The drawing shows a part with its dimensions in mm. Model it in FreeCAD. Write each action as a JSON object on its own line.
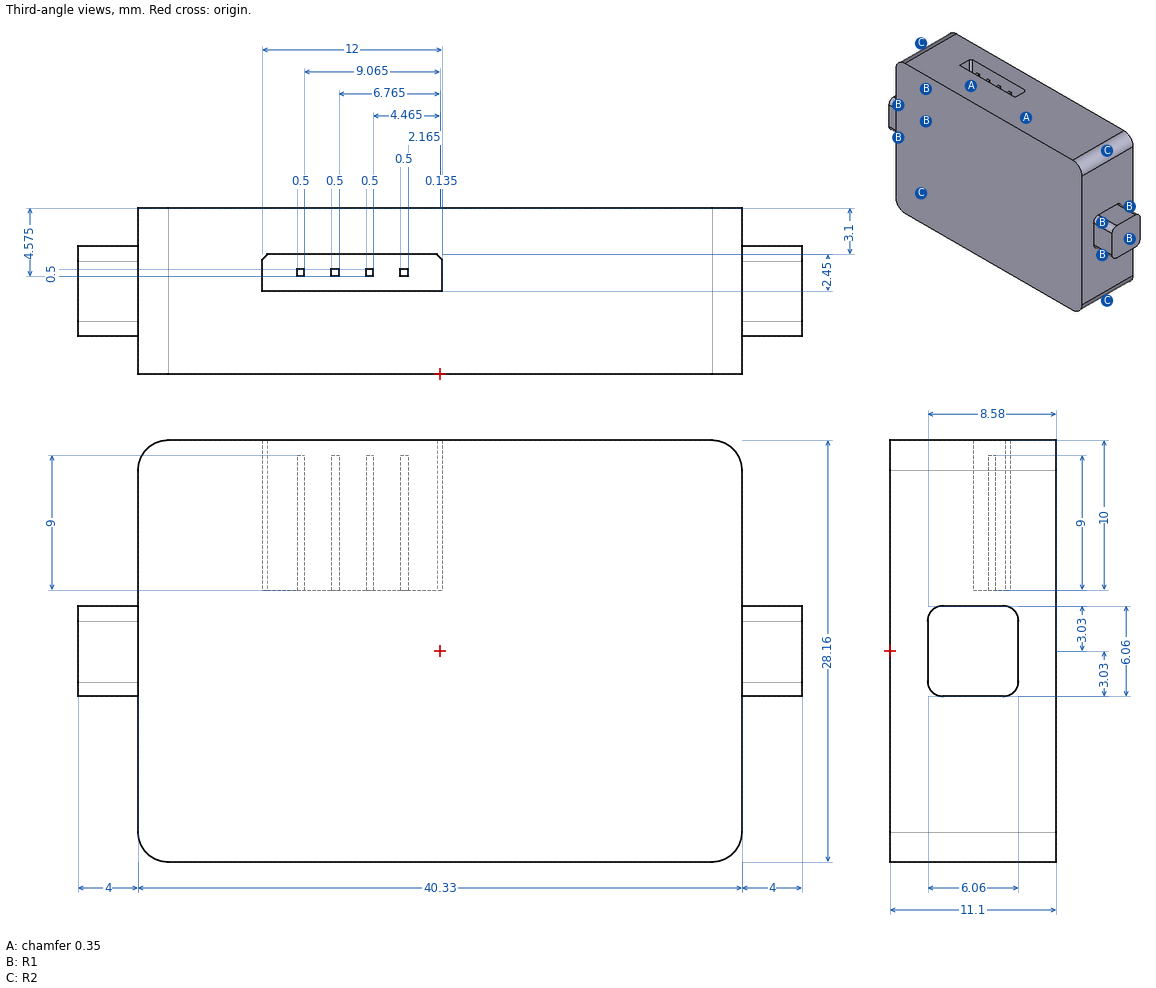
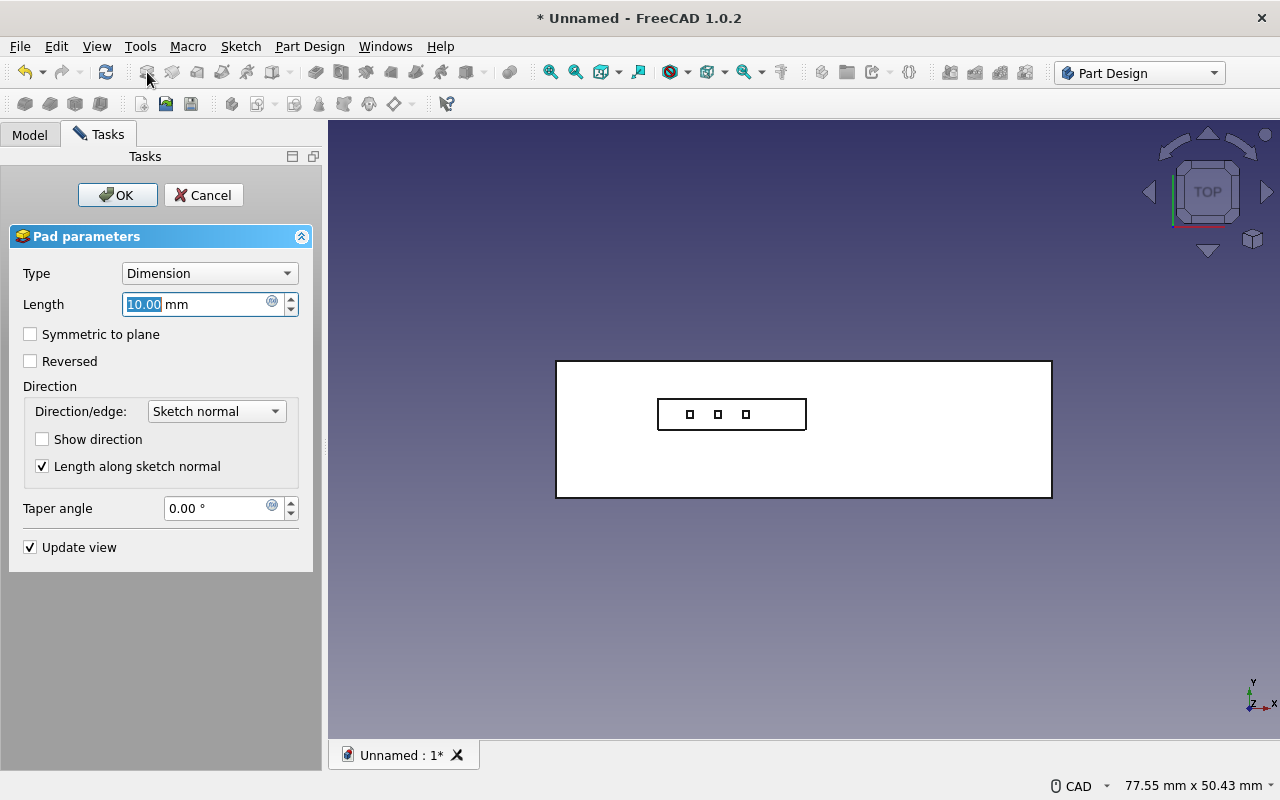
{"action": "type", "text": "9"}
{"action": "key", "text": "Tab"}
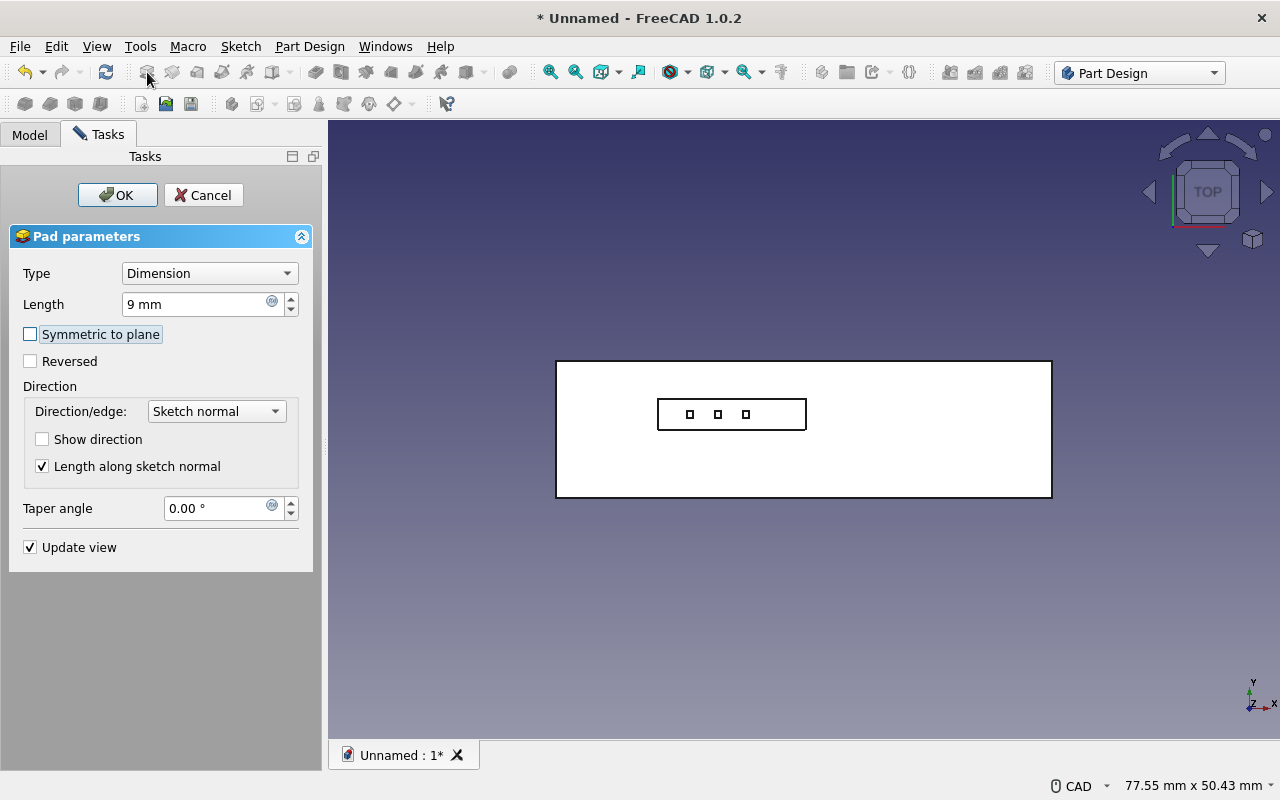
{"action": "left_click", "coordinate": [118, 195]}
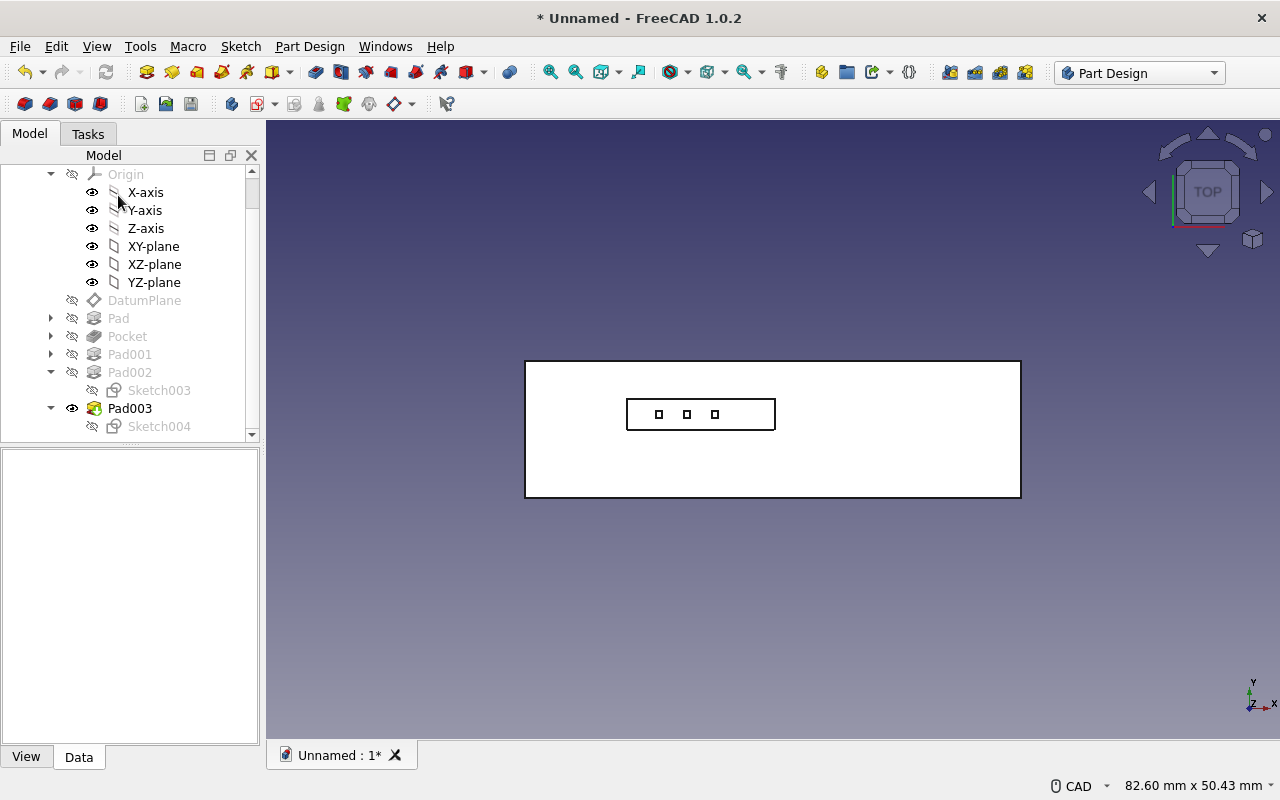
{"action": "left_click", "coordinate": [743, 413]}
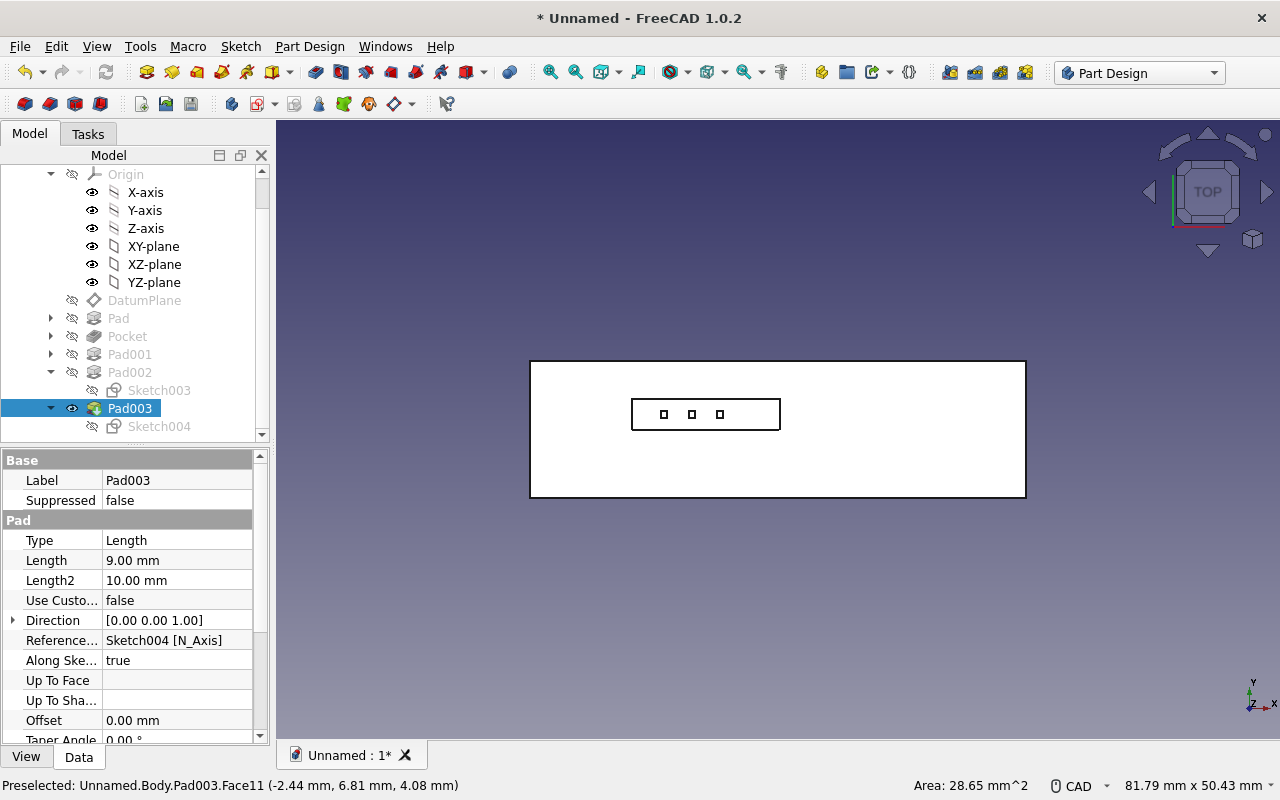
{"action": "left_click", "coordinate": [256, 104]}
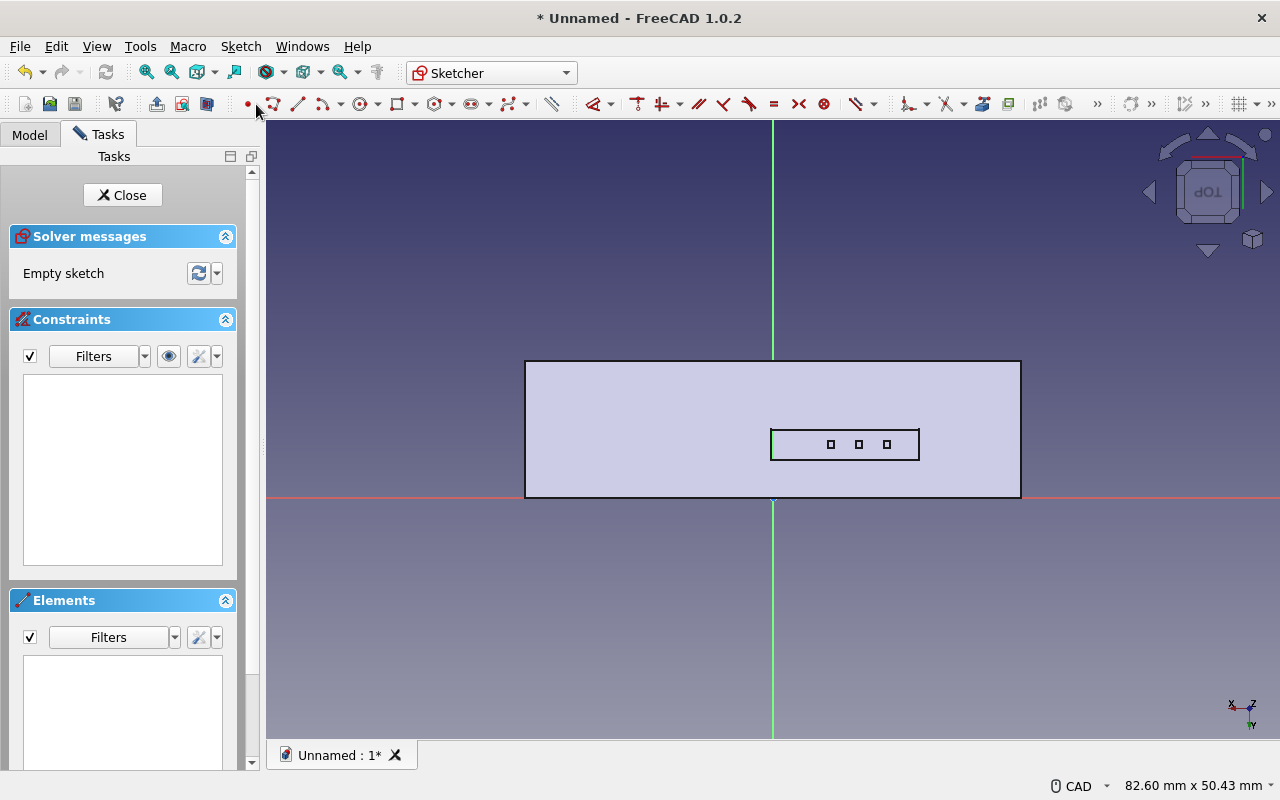
{"action": "left_click", "coordinate": [207, 104]}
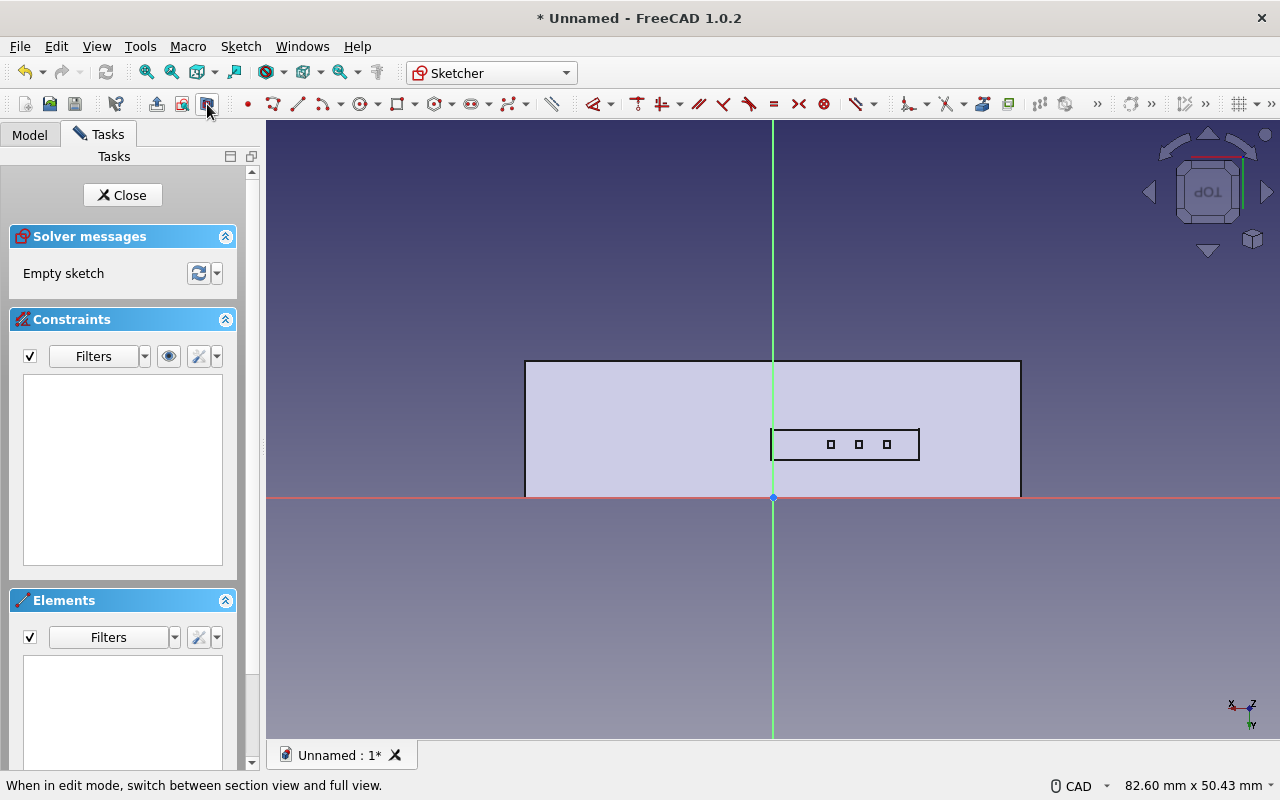
{"action": "scroll", "coordinate": [808, 445], "scroll_direction": "up", "scroll_amount": 15}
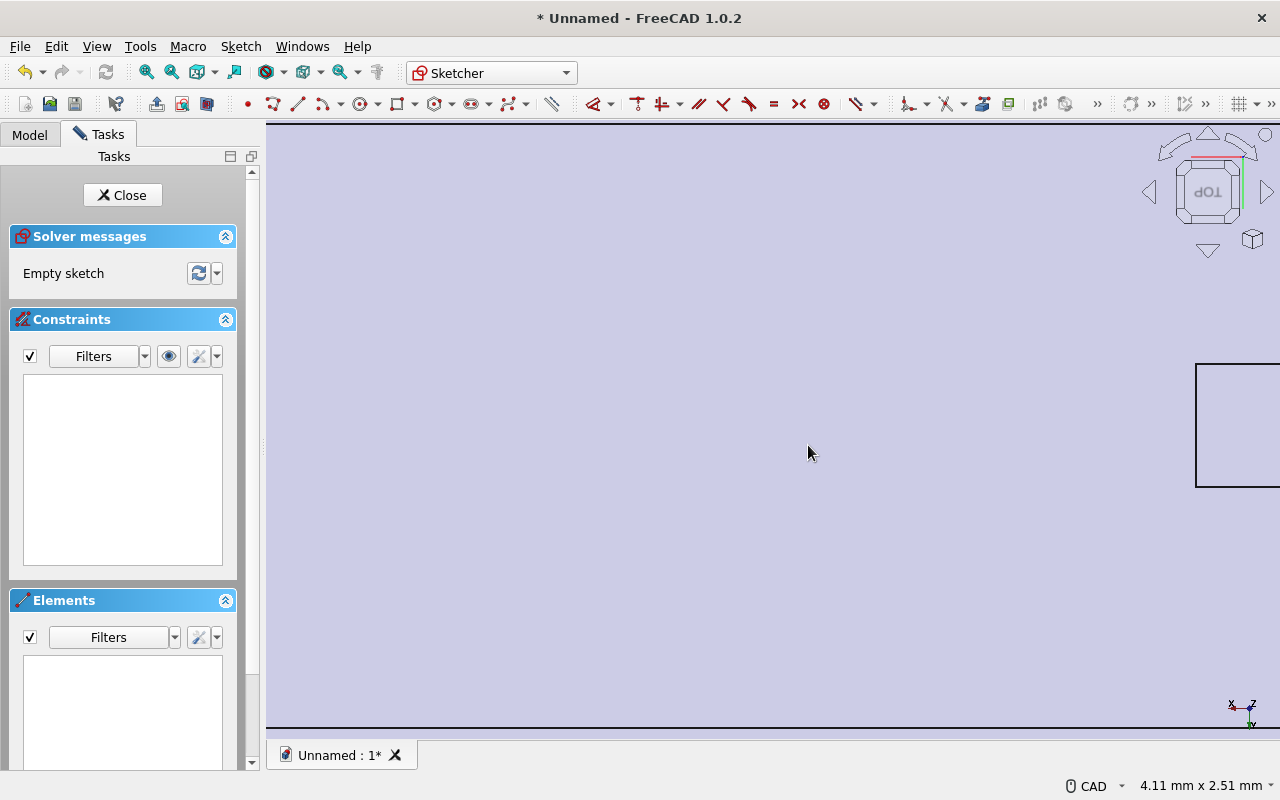
{"action": "scroll", "coordinate": [684, 424], "scroll_direction": "up", "scroll_amount": 6}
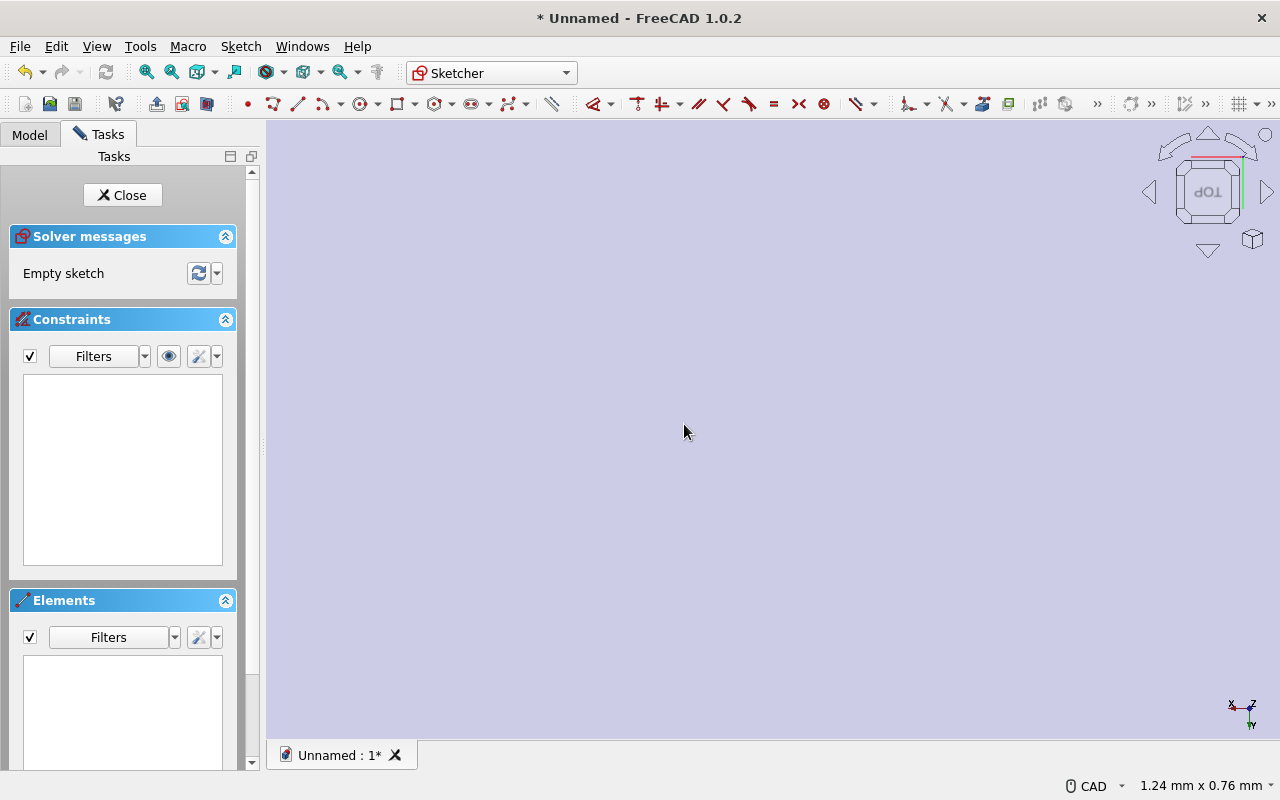
{"action": "left_click", "coordinate": [396, 104]}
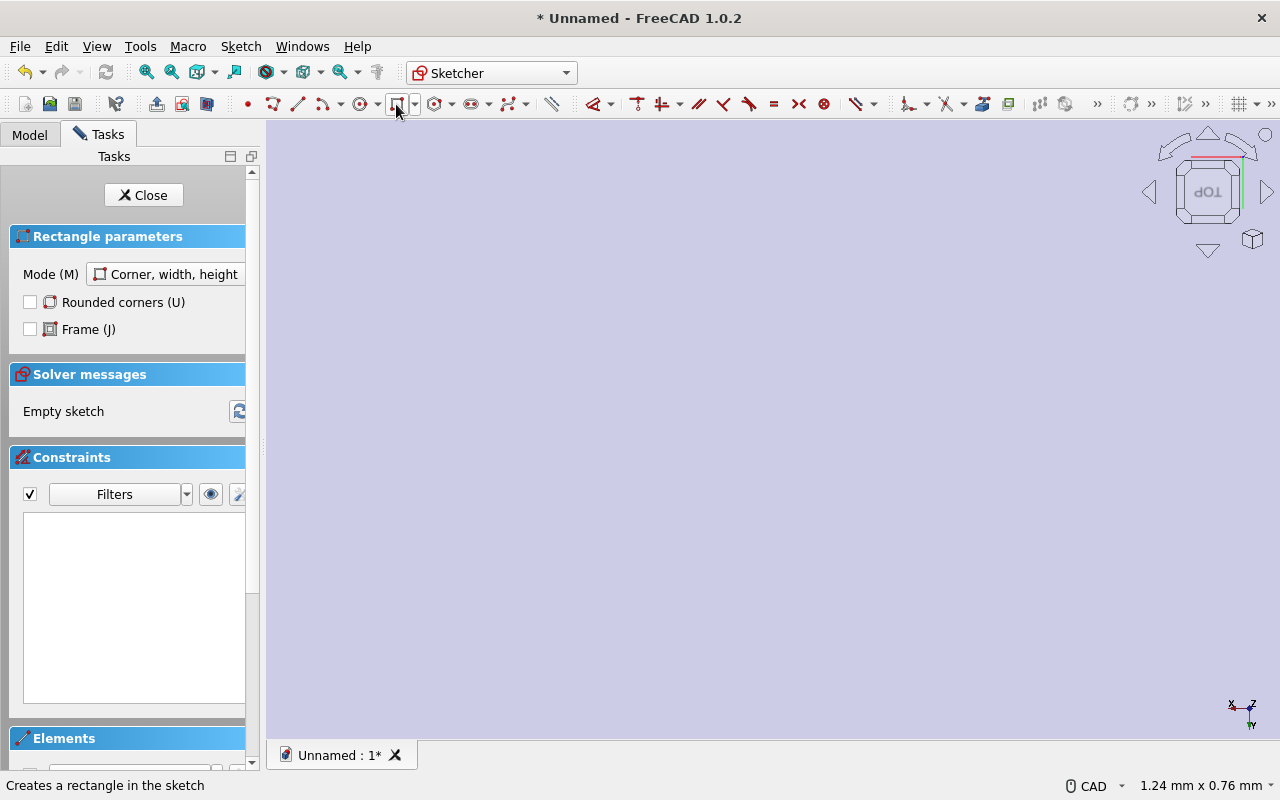
{"action": "left_click", "coordinate": [499, 224]}
{"action": "mouse_move", "coordinate": [908, 633]}